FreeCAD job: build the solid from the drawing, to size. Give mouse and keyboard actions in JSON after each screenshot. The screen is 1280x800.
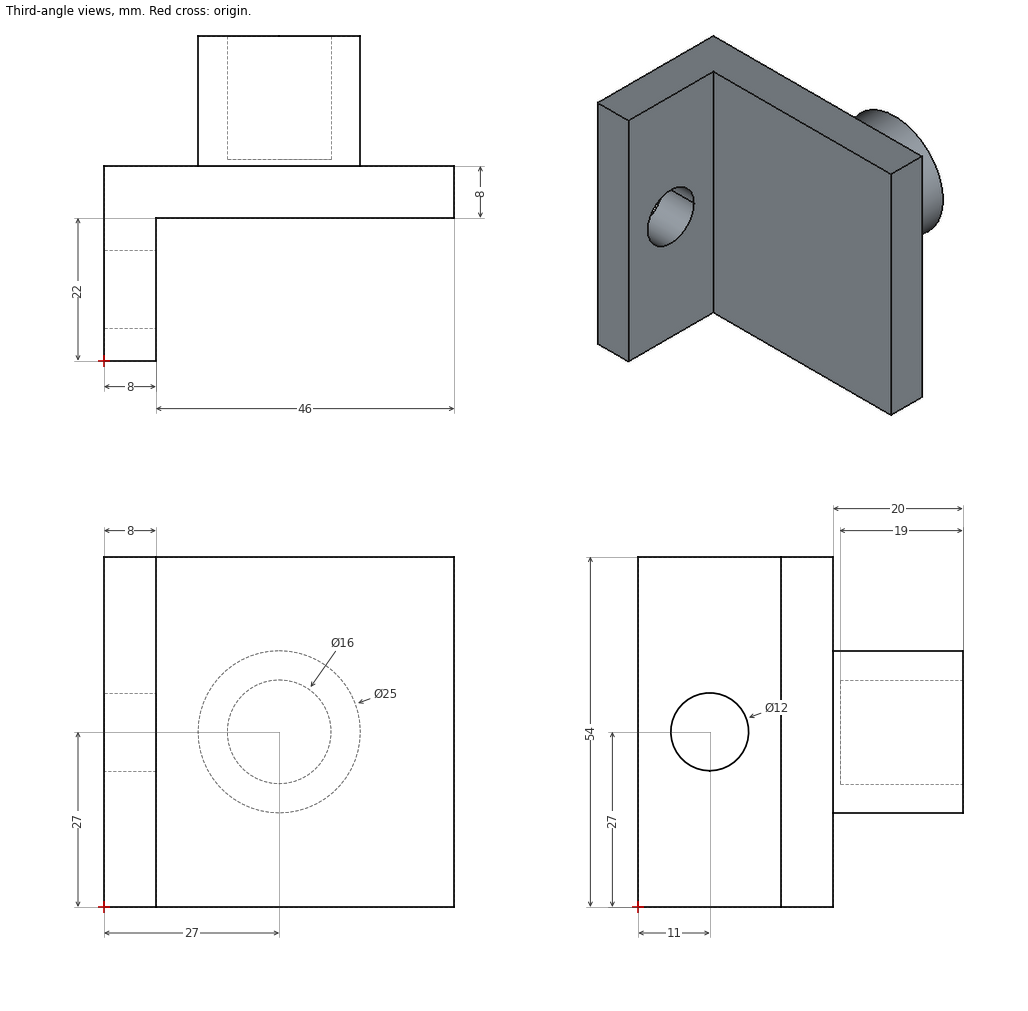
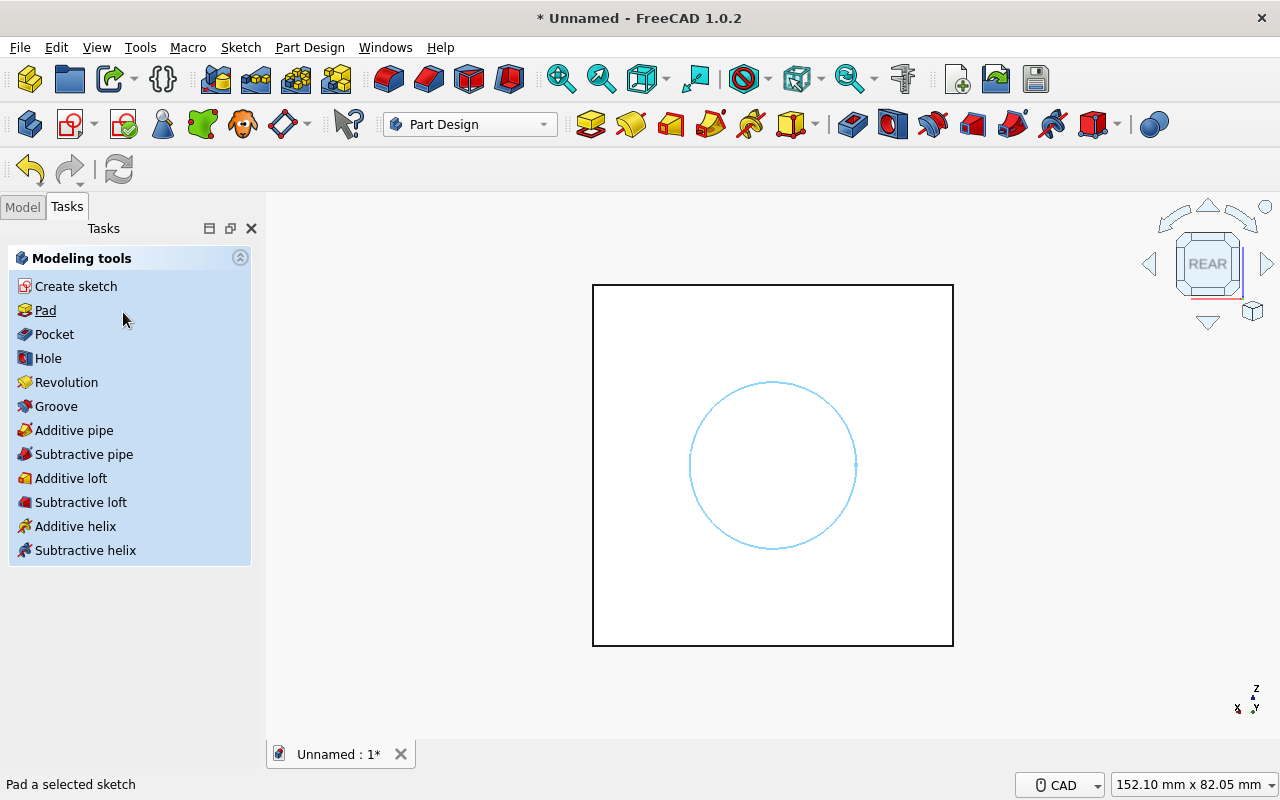
{"action": "left_click", "coordinate": [592, 124]}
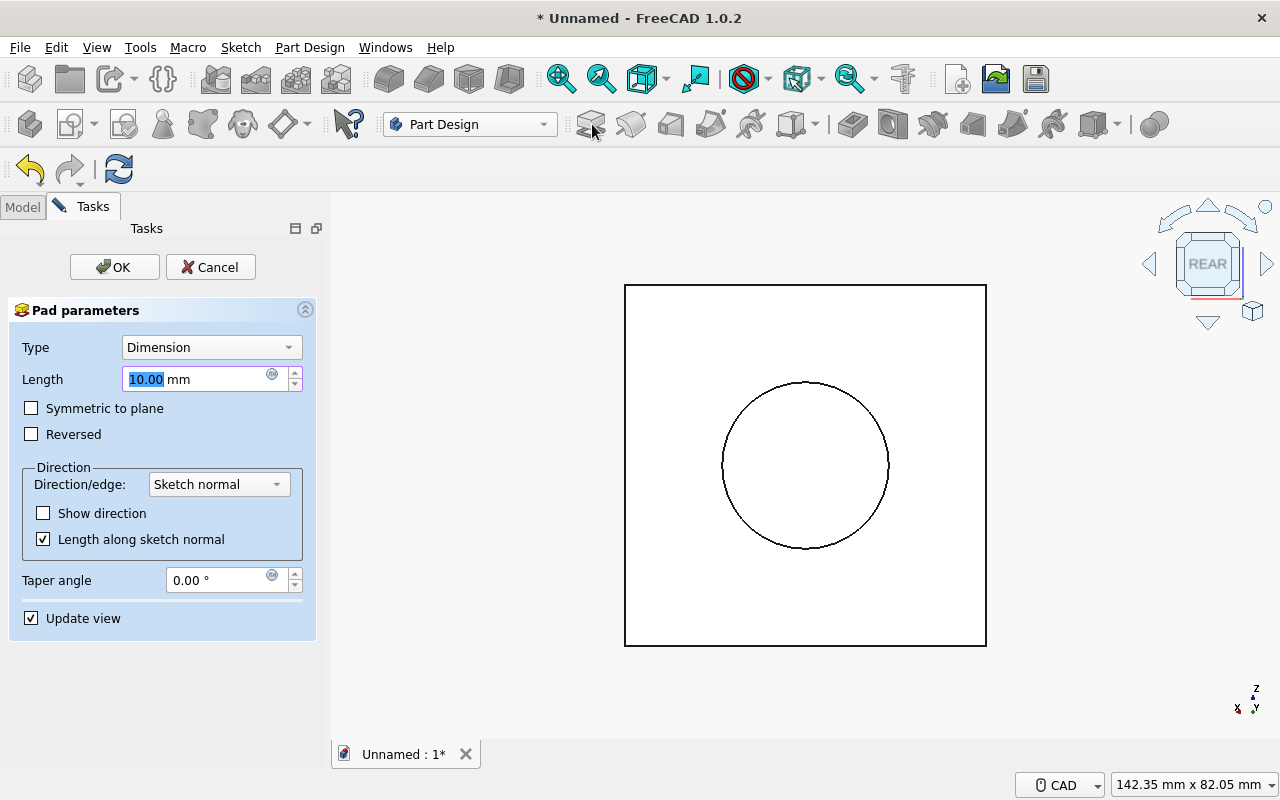
{"action": "type", "text": "20"}
{"action": "key", "text": "Tab"}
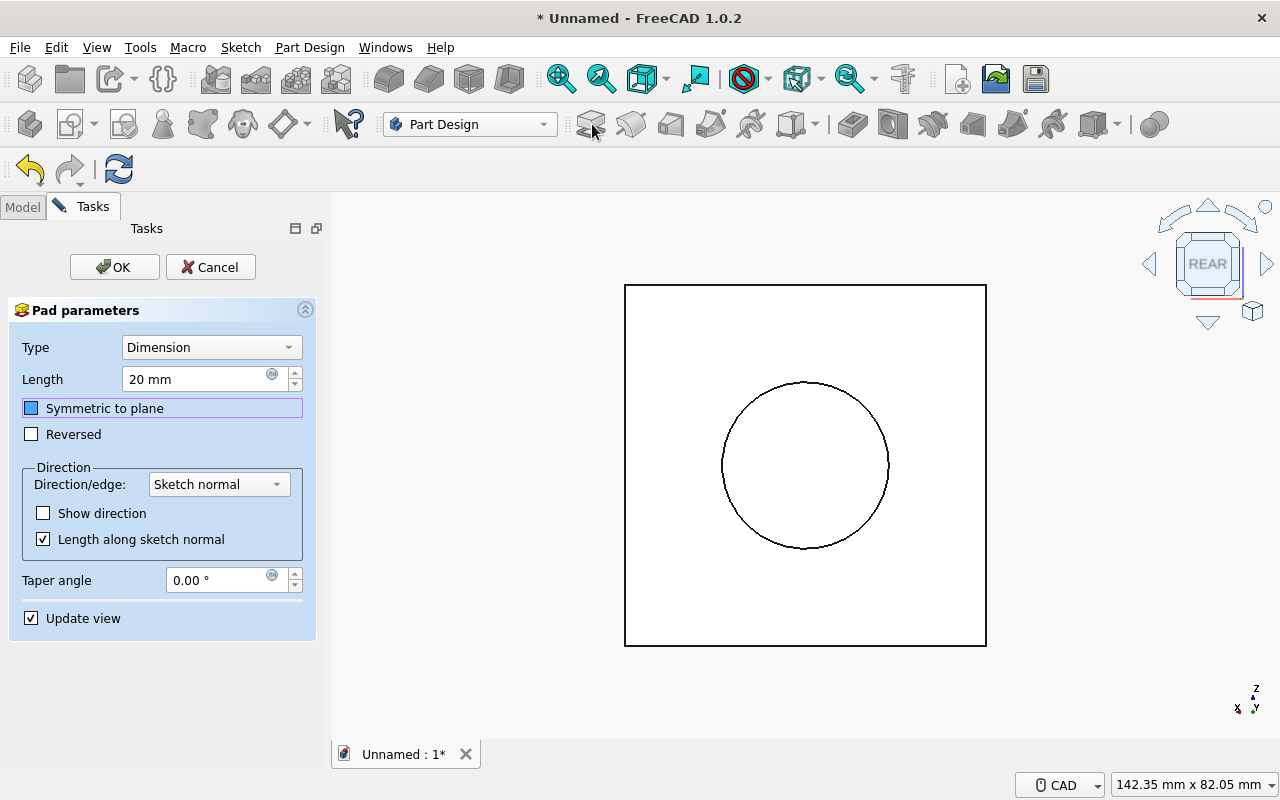
{"action": "left_click", "coordinate": [115, 267]}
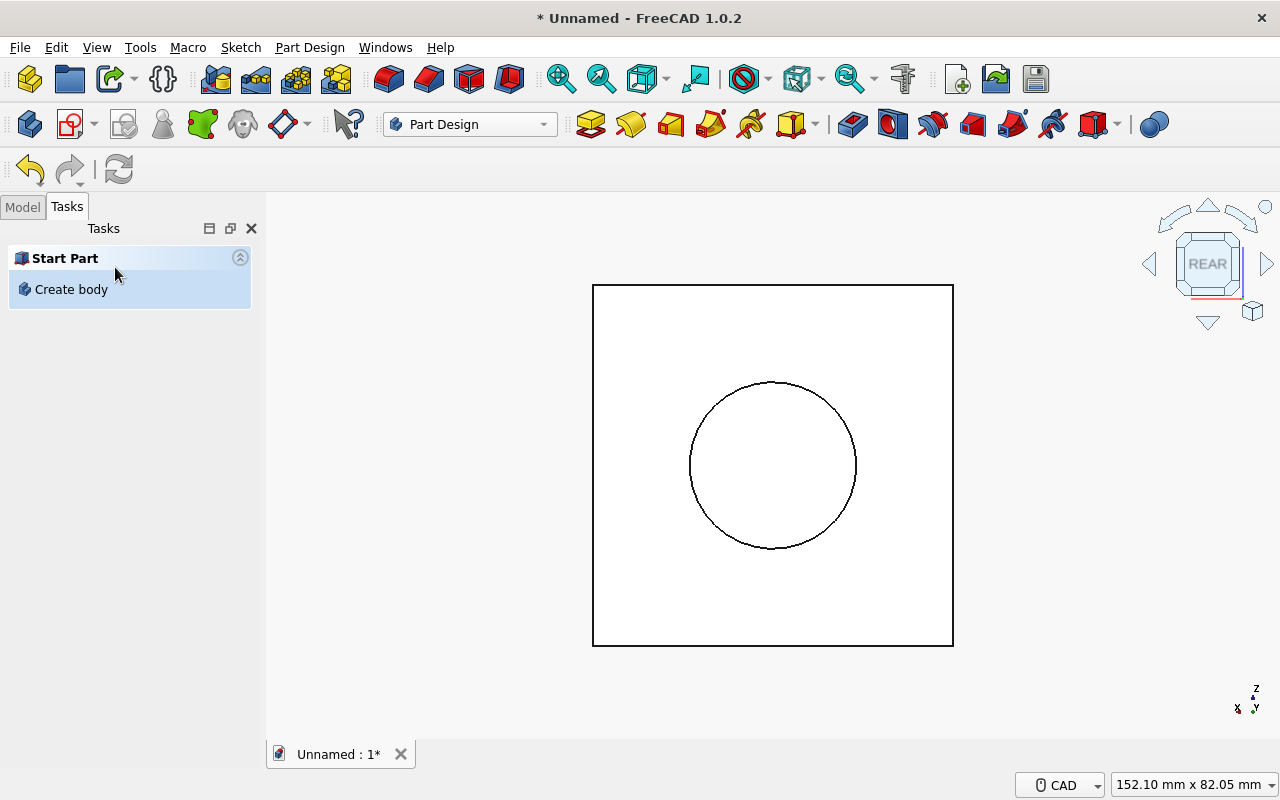
{"action": "left_click", "coordinate": [773, 465]}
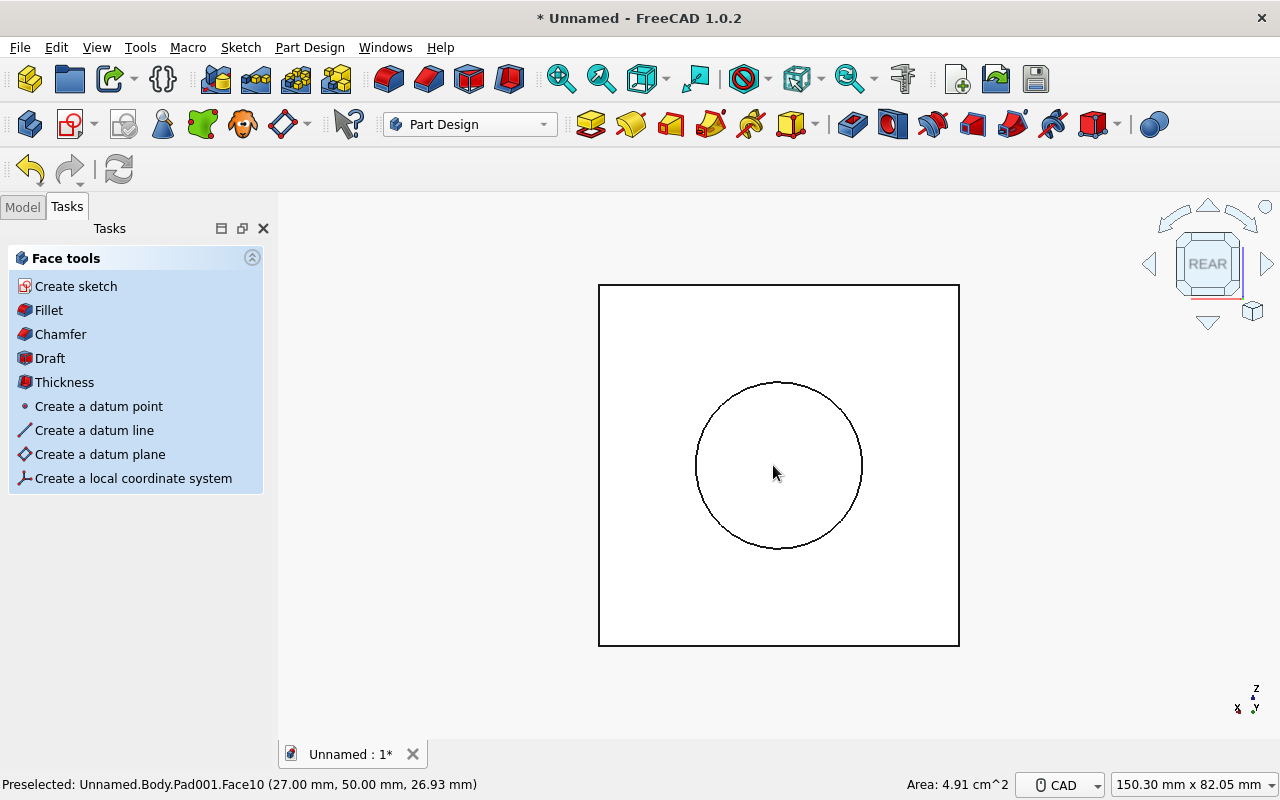
{"action": "left_click", "coordinate": [70, 124]}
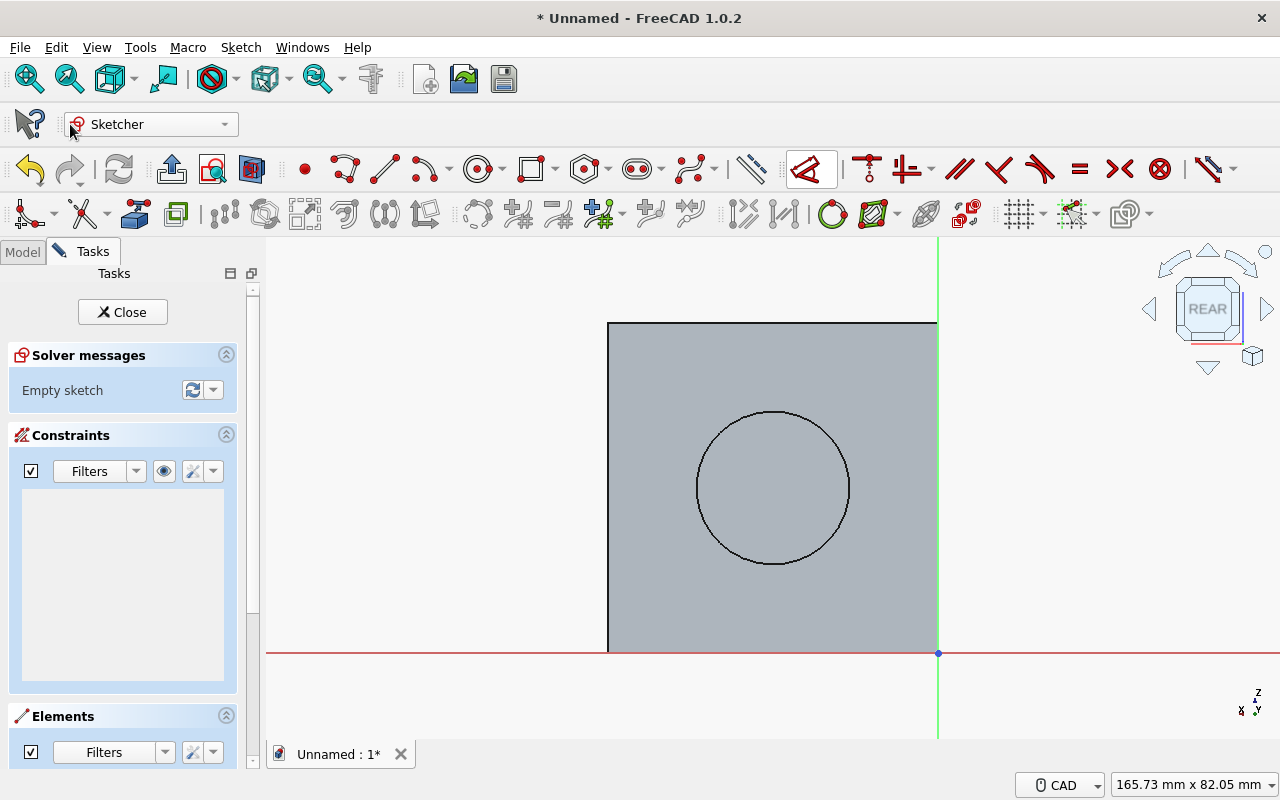
{"action": "scroll", "coordinate": [1089, 664], "scroll_direction": "up", "scroll_amount": 2}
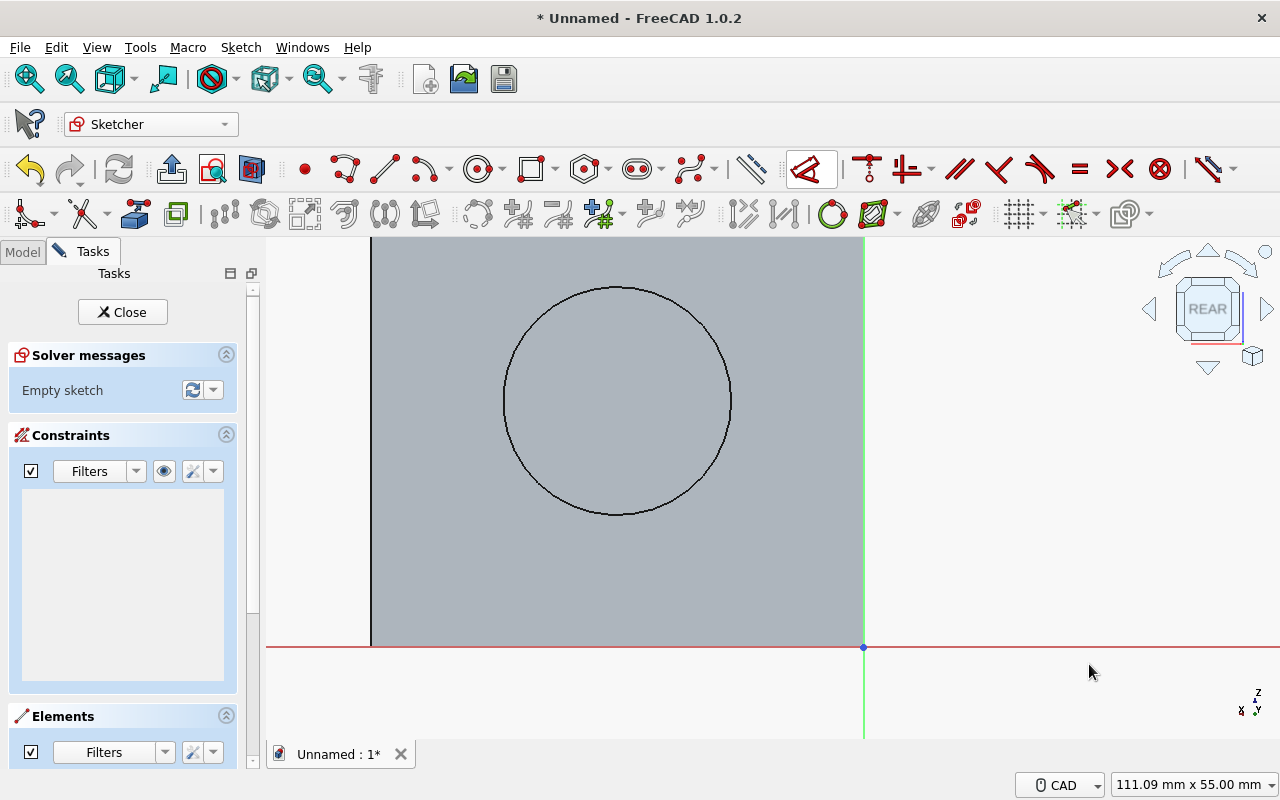
{"action": "left_click", "coordinate": [478, 170]}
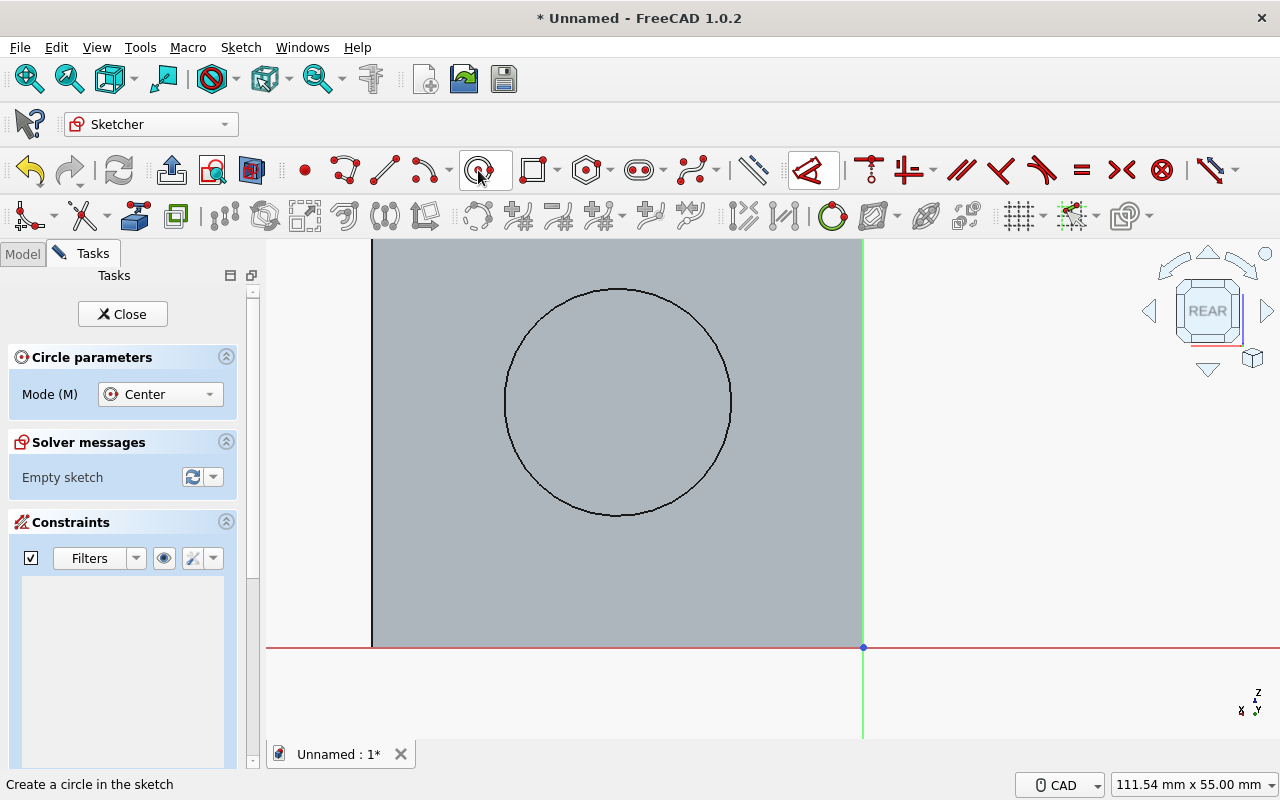
{"action": "left_click", "coordinate": [618, 402]}
{"action": "mouse_move", "coordinate": [669, 351]}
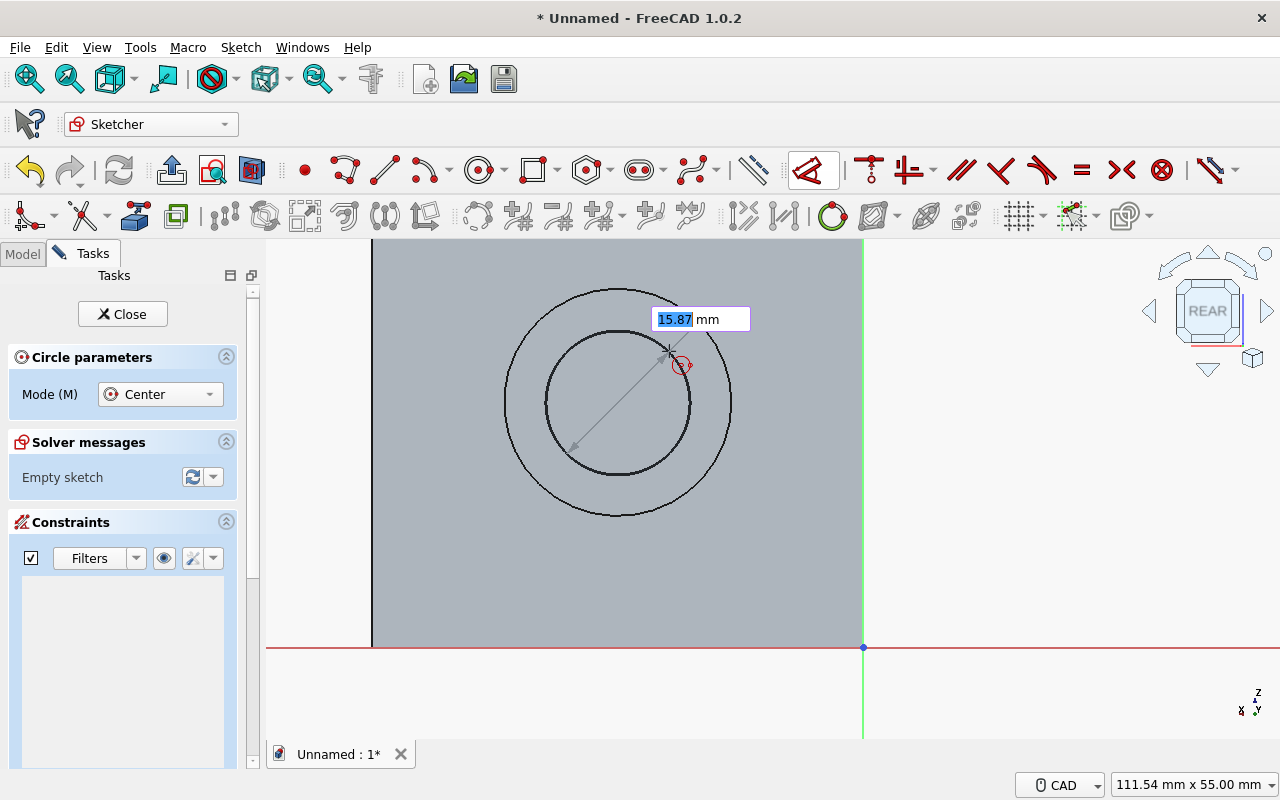
{"action": "type", "text": "16"}
{"action": "key", "text": "Return"}
{"action": "key", "text": "Escape"}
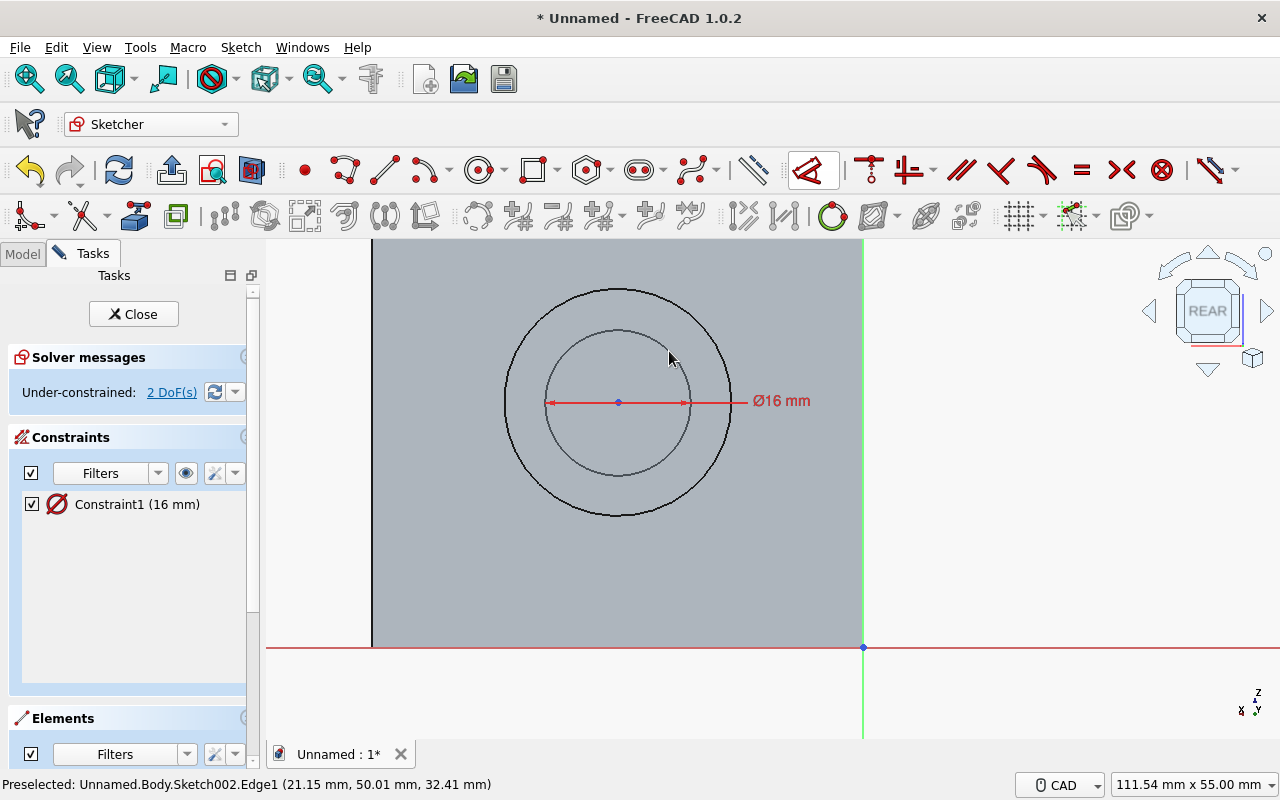
{"action": "left_click", "coordinate": [618, 403]}